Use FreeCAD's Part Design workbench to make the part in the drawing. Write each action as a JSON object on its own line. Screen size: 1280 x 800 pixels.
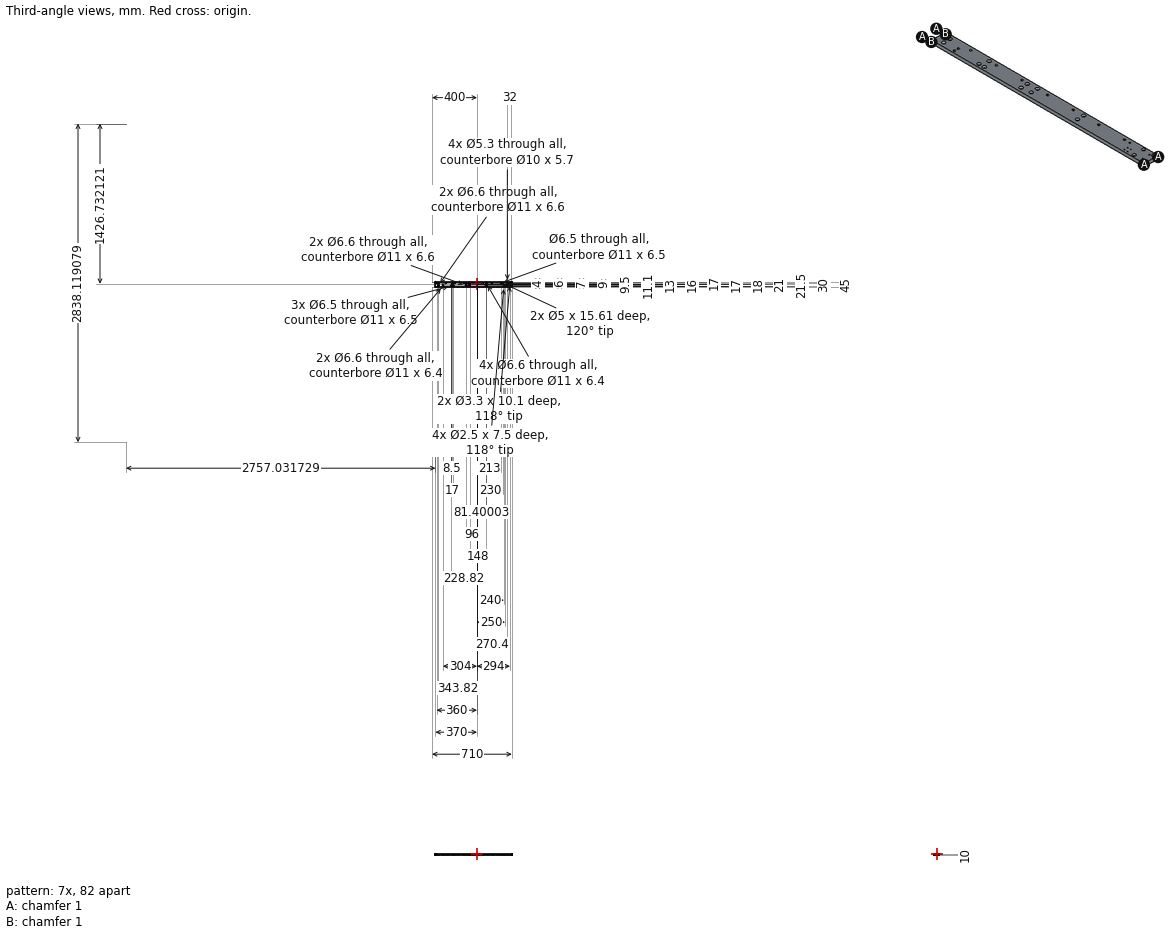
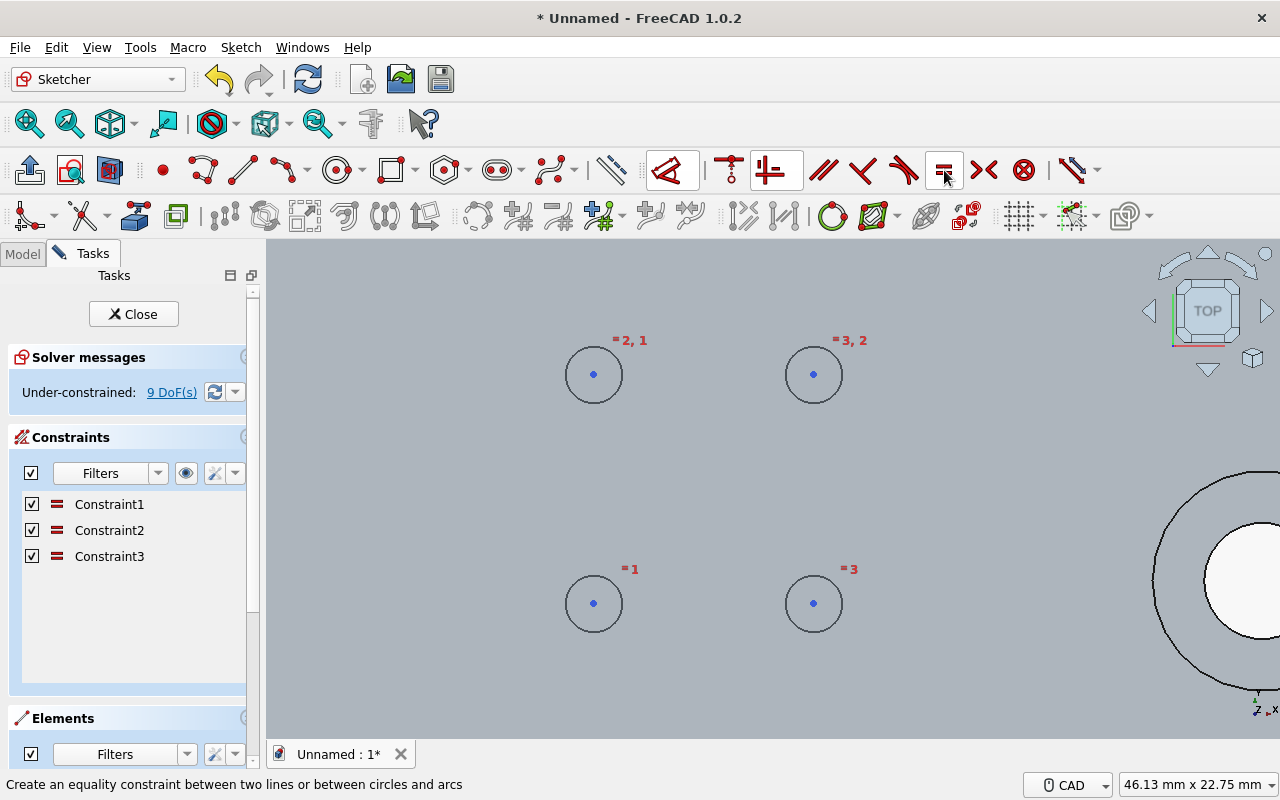
{"action": "left_click", "coordinate": [594, 604]}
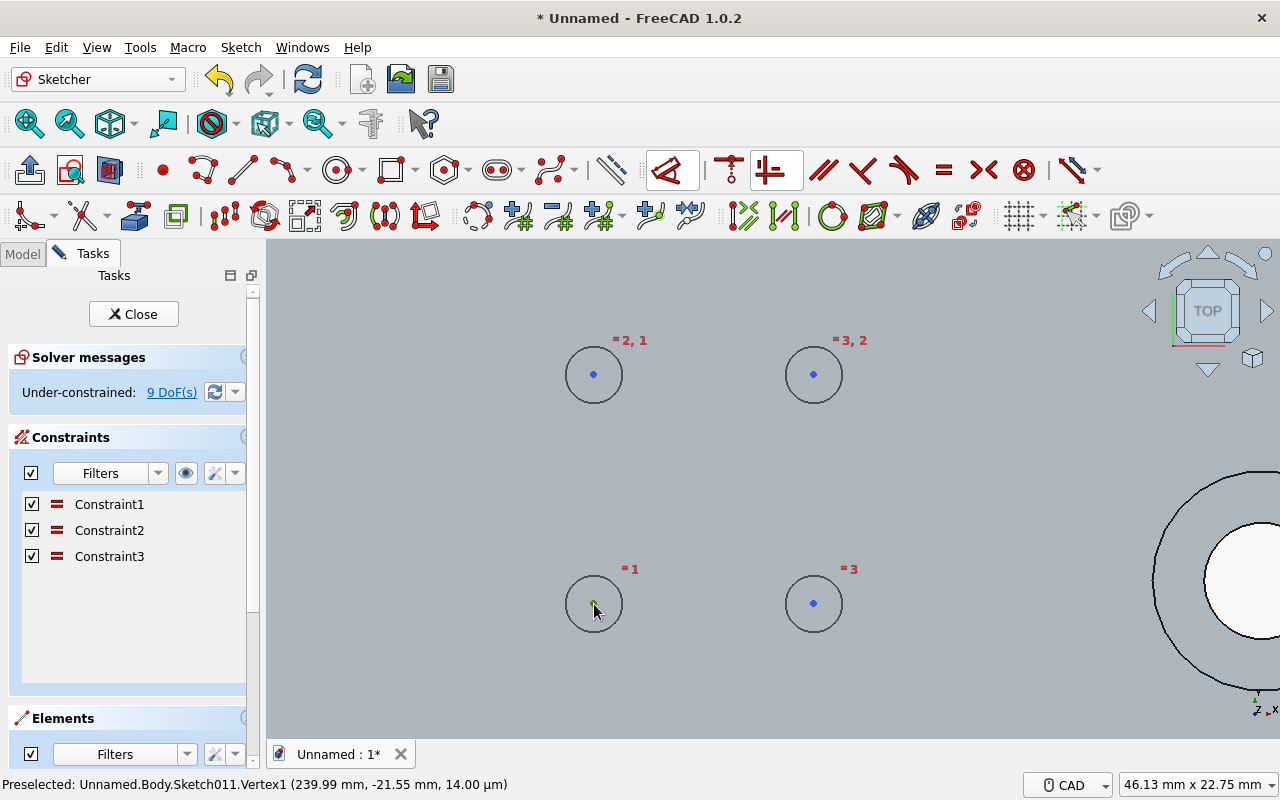
{"action": "left_click", "coordinate": [594, 375]}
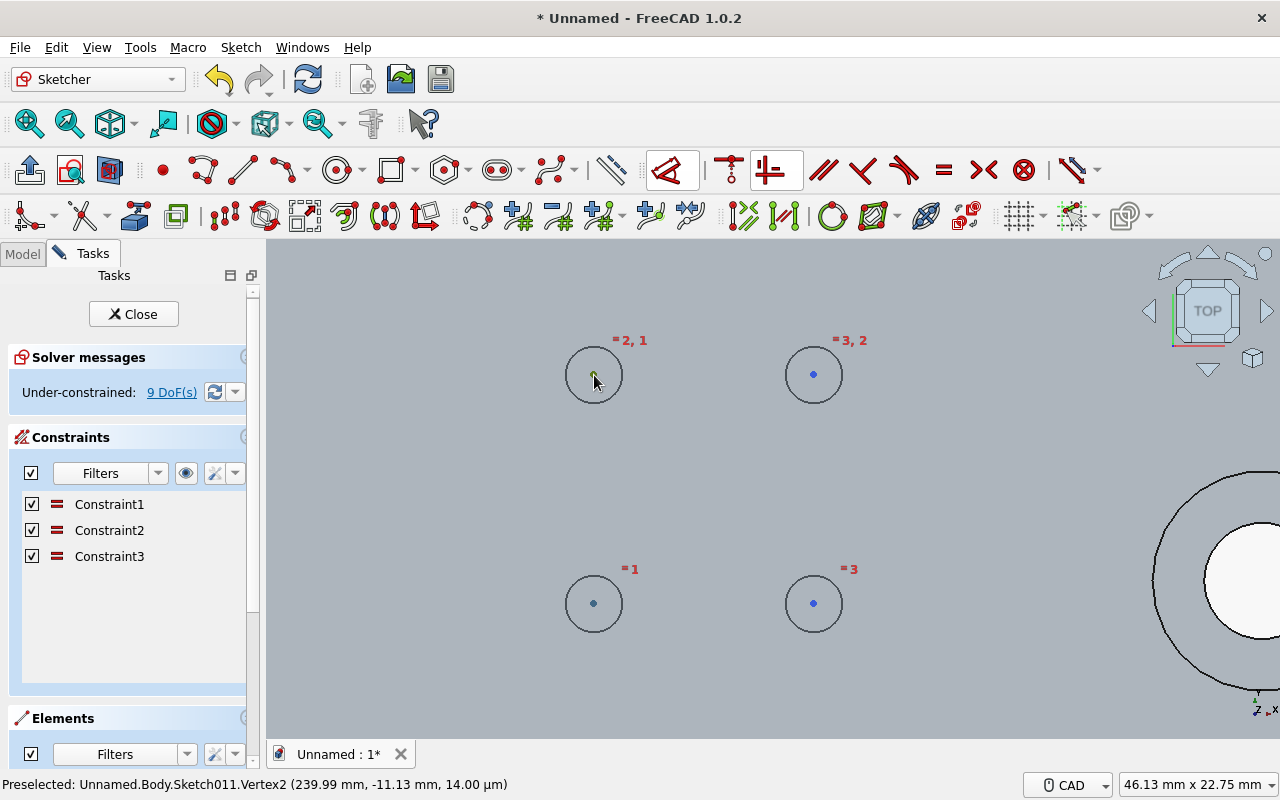
{"action": "left_click", "coordinate": [798, 170]}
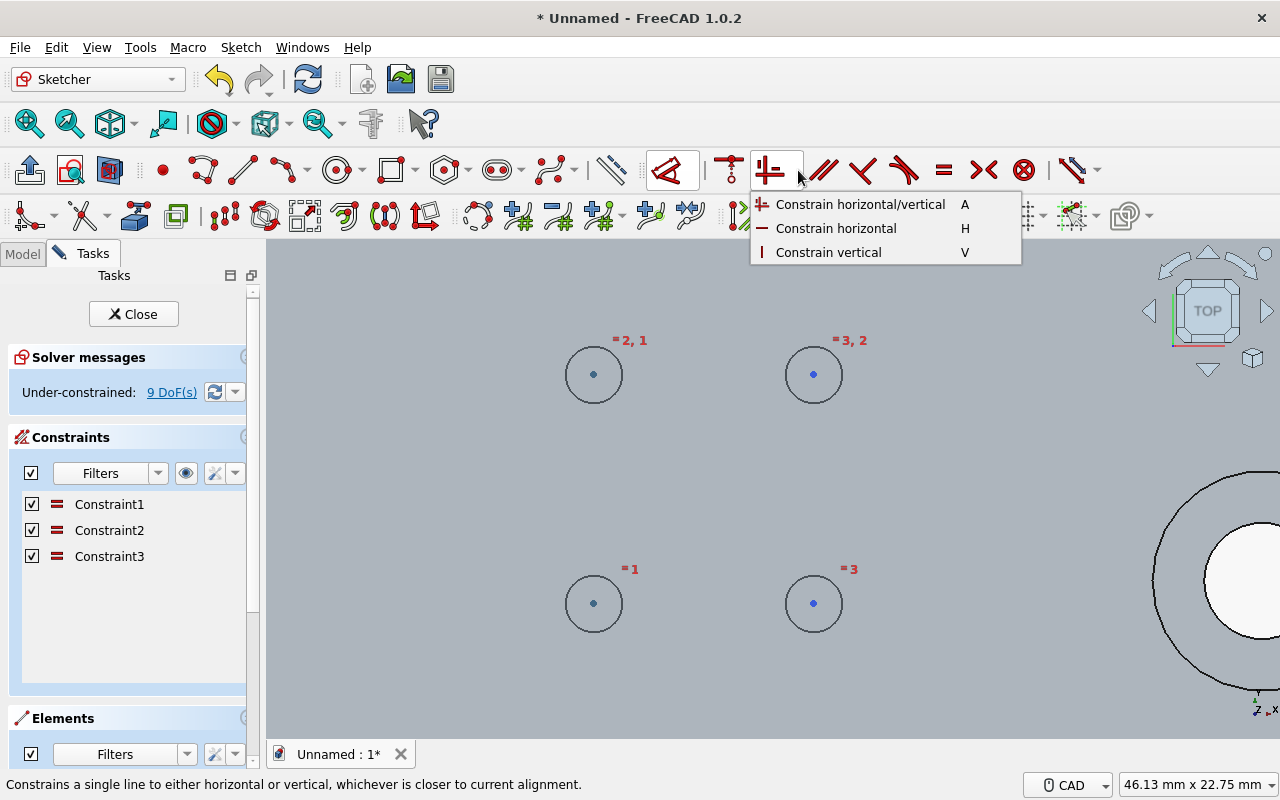
{"action": "left_click", "coordinate": [886, 252]}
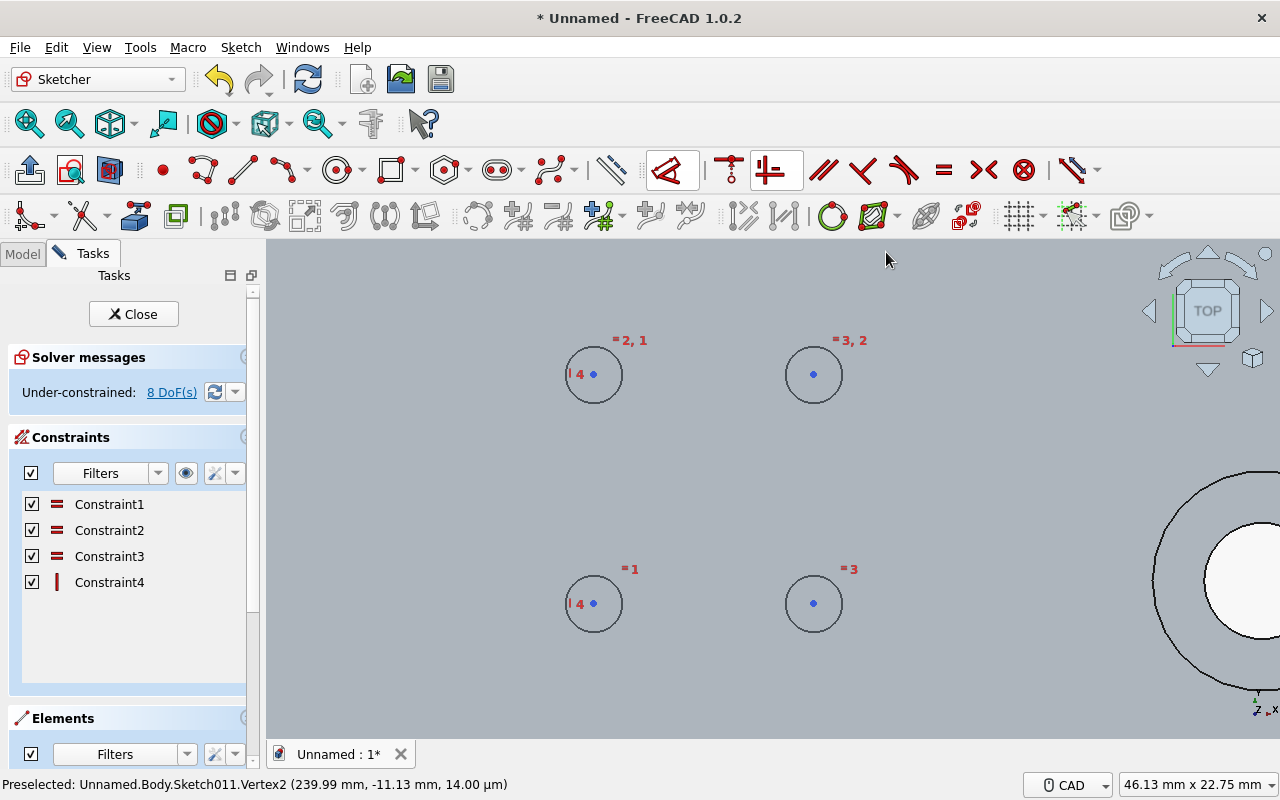
{"action": "left_click", "coordinate": [594, 375]}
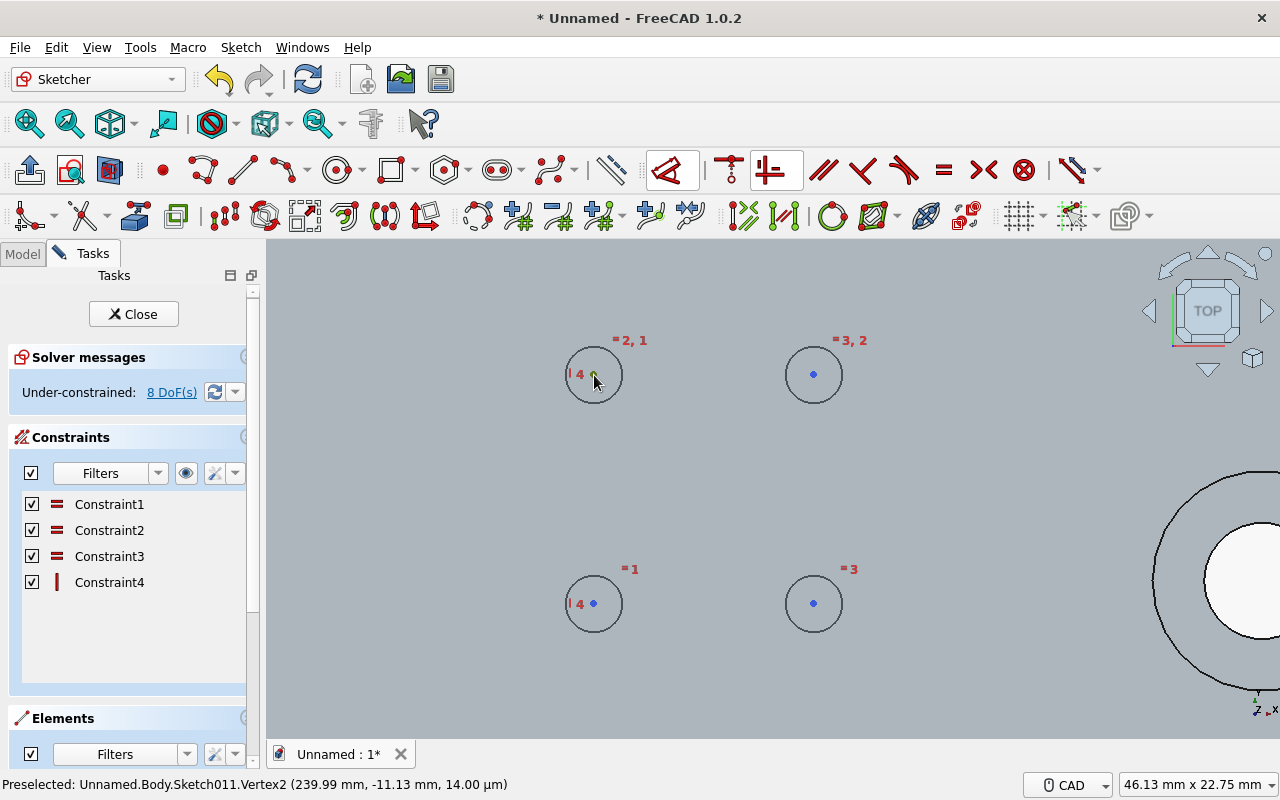
{"action": "left_click", "coordinate": [814, 375]}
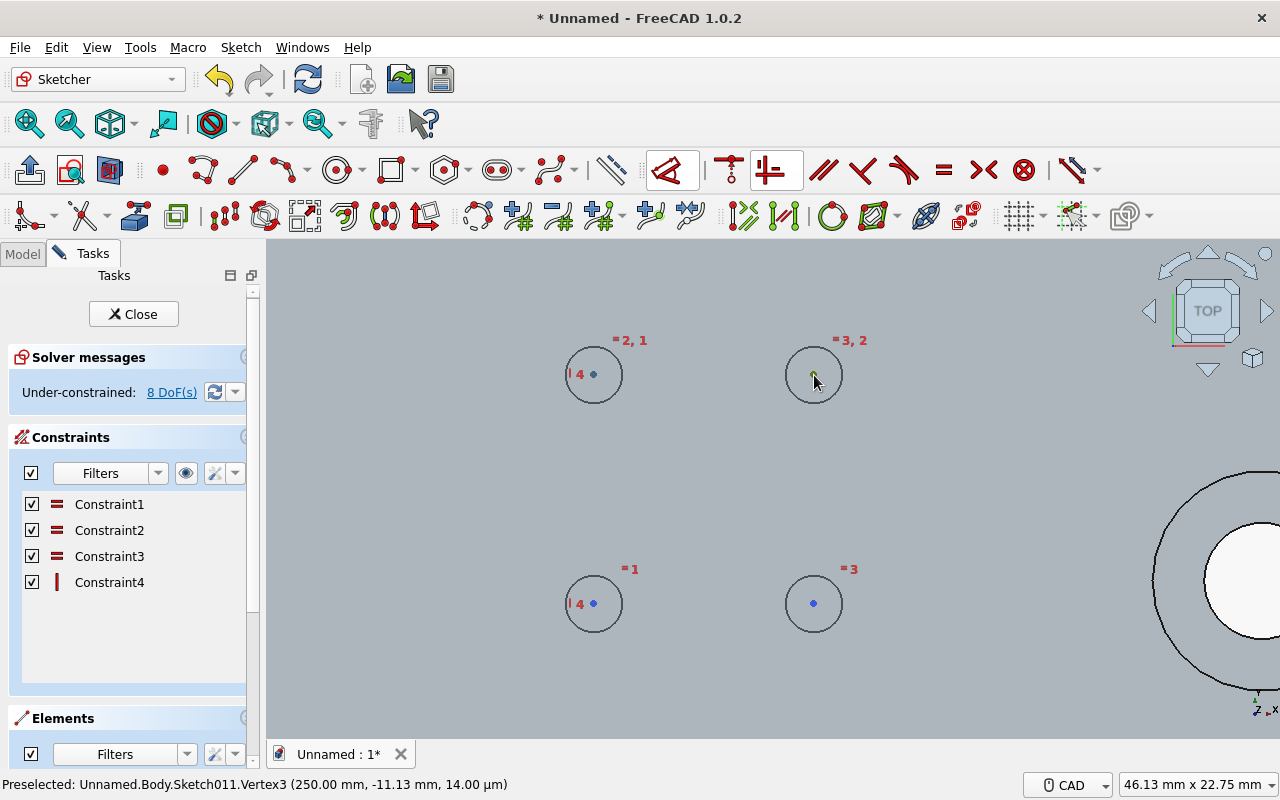
{"action": "left_click", "coordinate": [798, 170]}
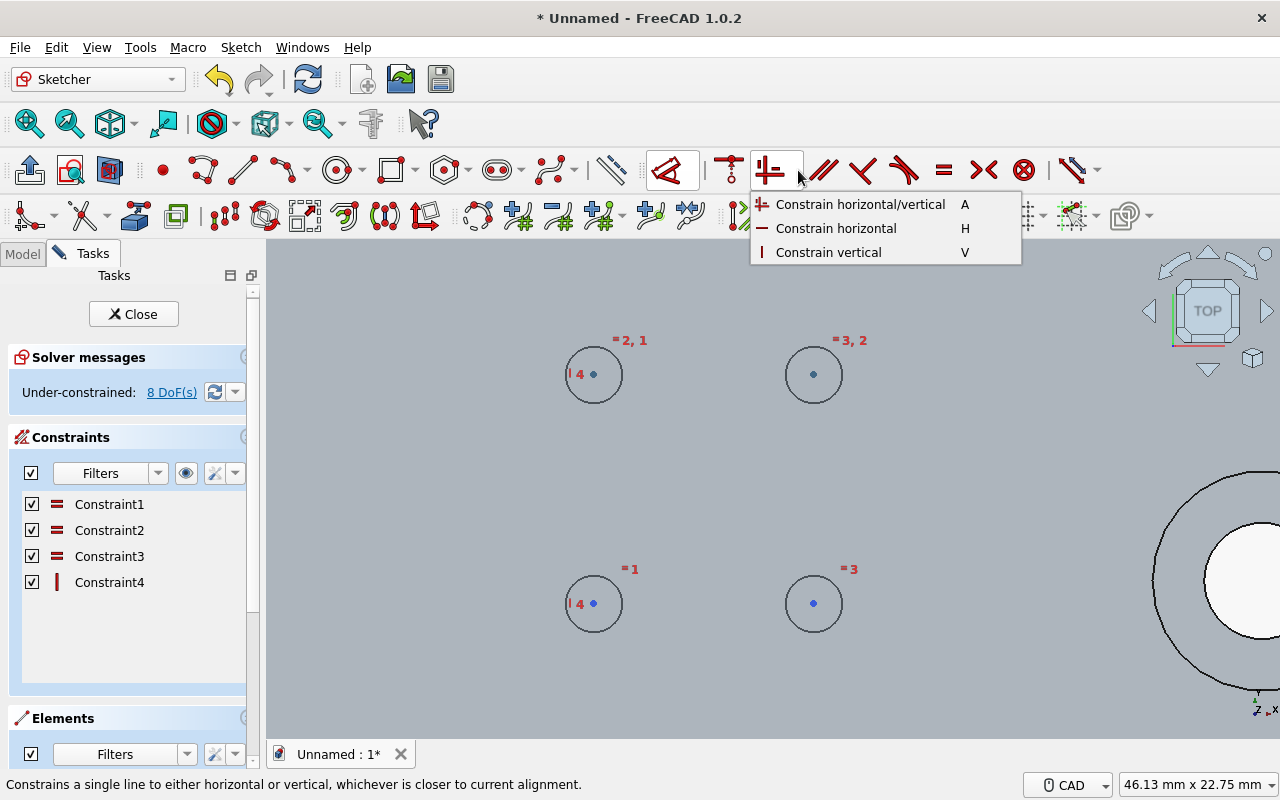
{"action": "left_click", "coordinate": [886, 228]}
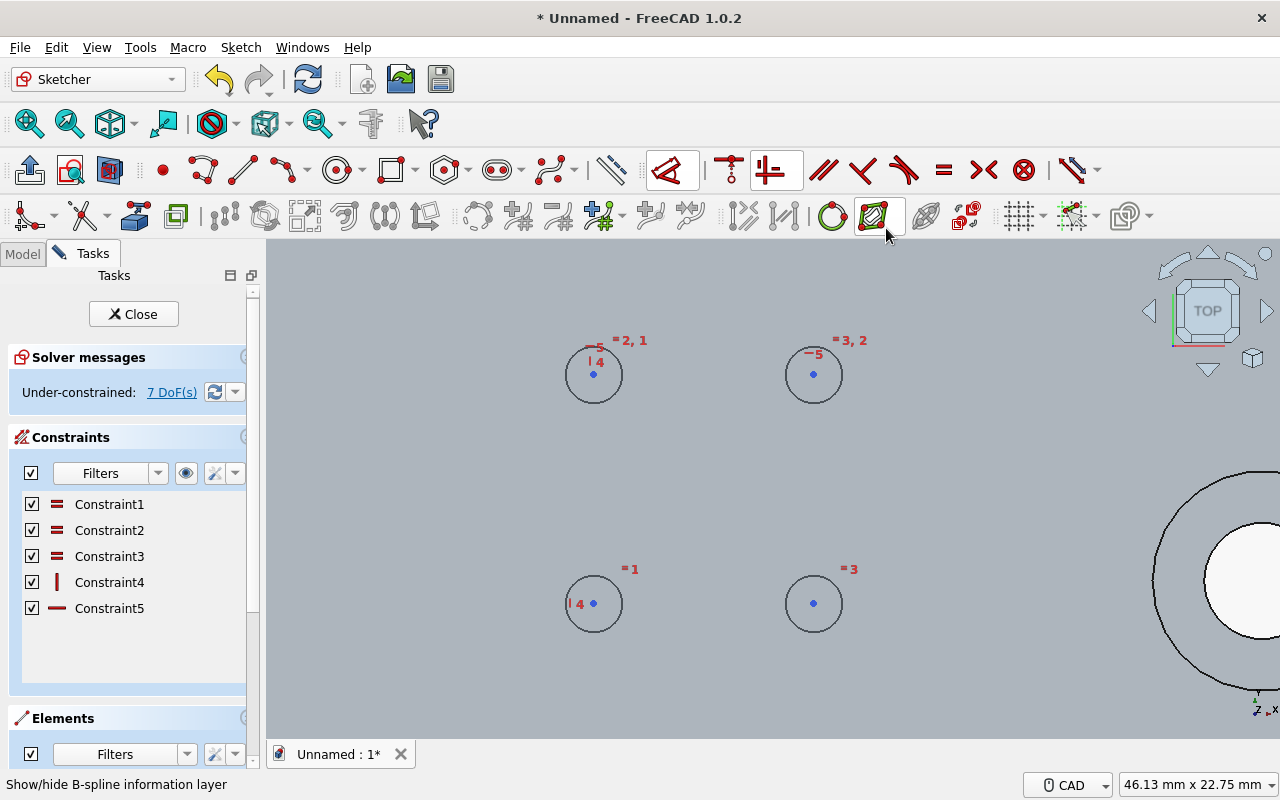
{"action": "left_click", "coordinate": [814, 375]}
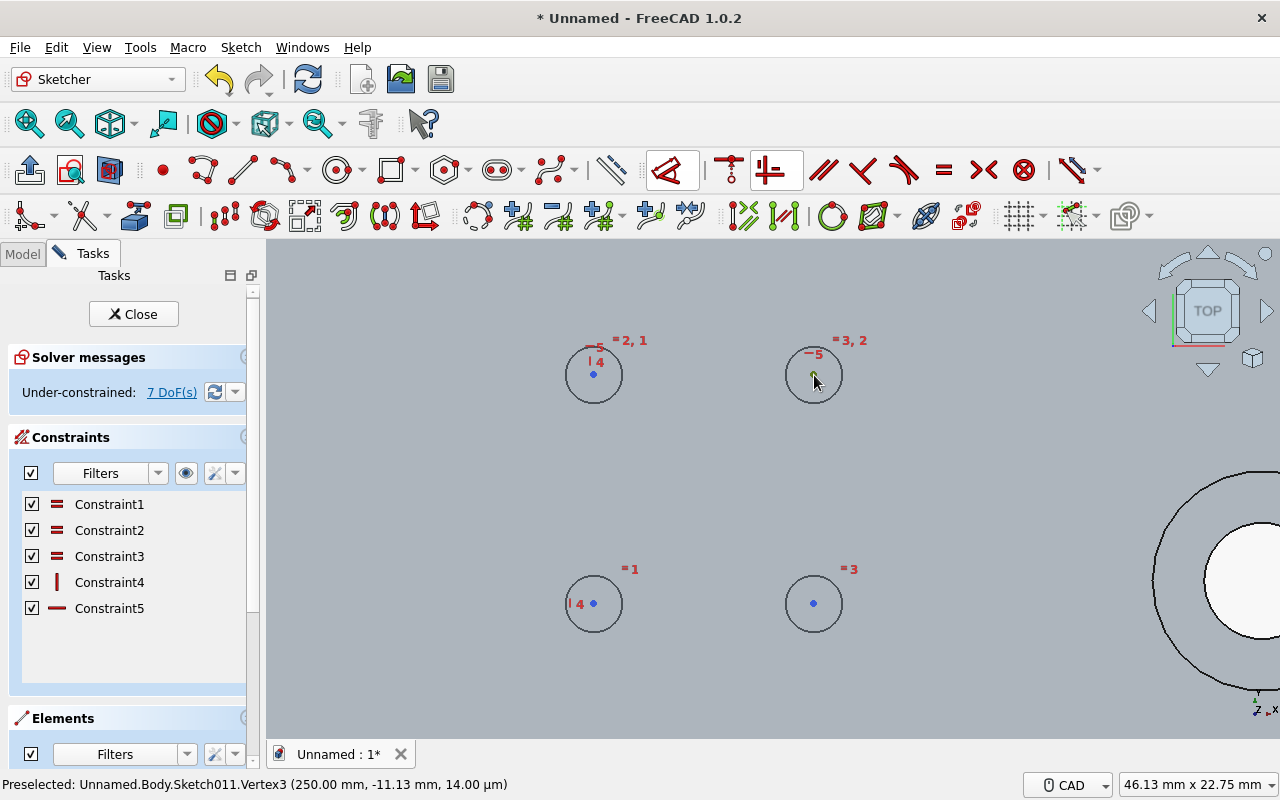
{"action": "left_click", "coordinate": [814, 604]}